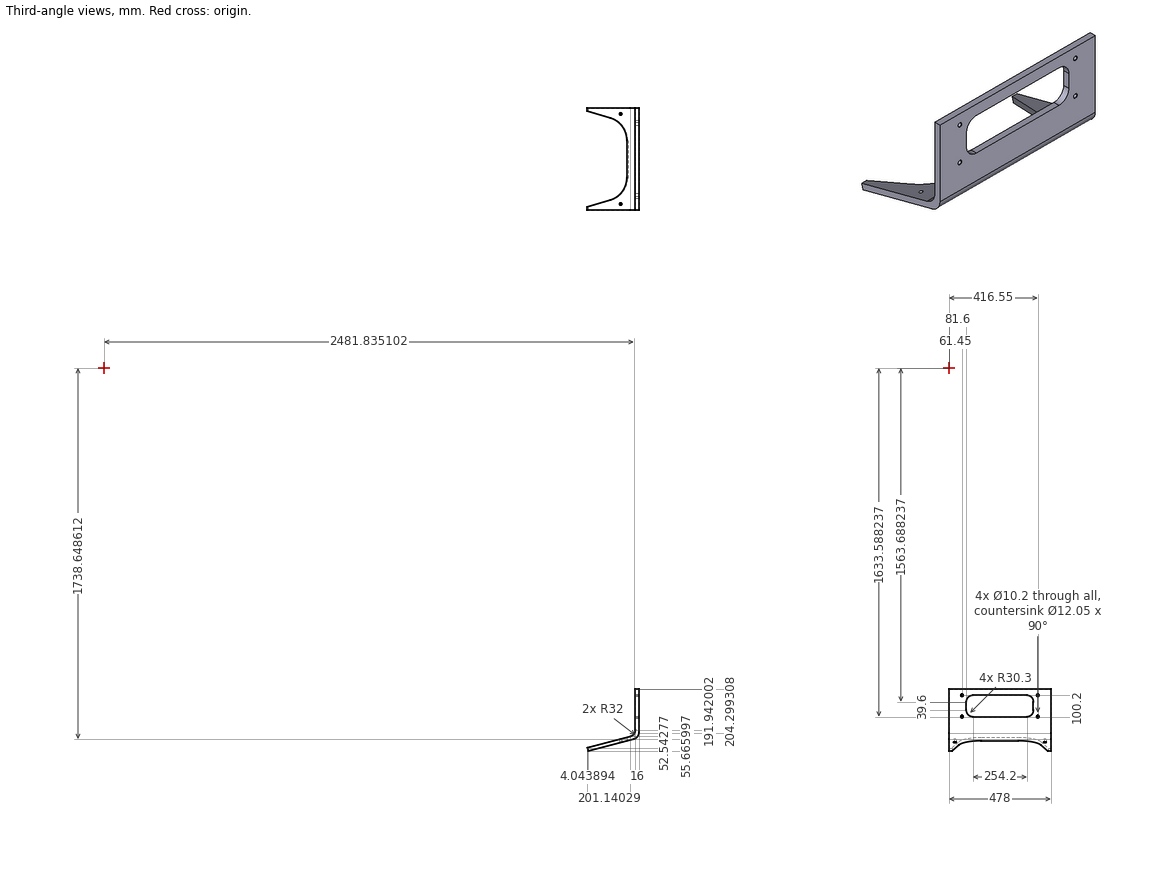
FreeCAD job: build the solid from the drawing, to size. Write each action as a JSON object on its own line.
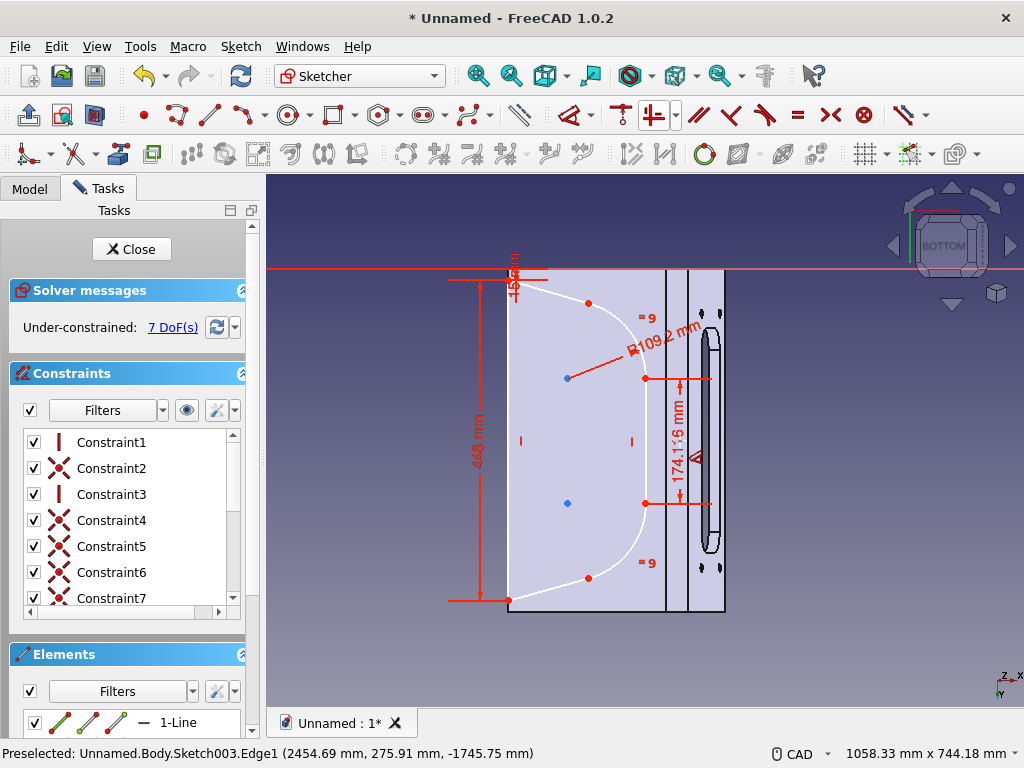
{"action": "left_click", "coordinate": [588, 303]}
{"action": "left_click", "coordinate": [622, 286]}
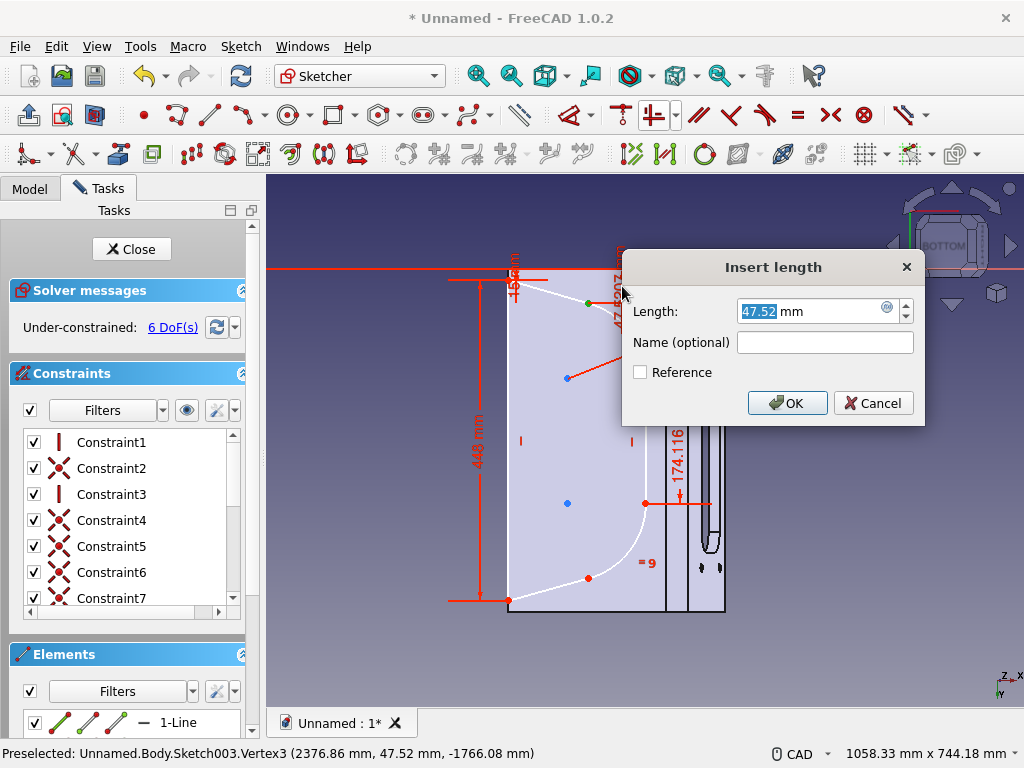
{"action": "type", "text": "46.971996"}
{"action": "key", "text": "Return"}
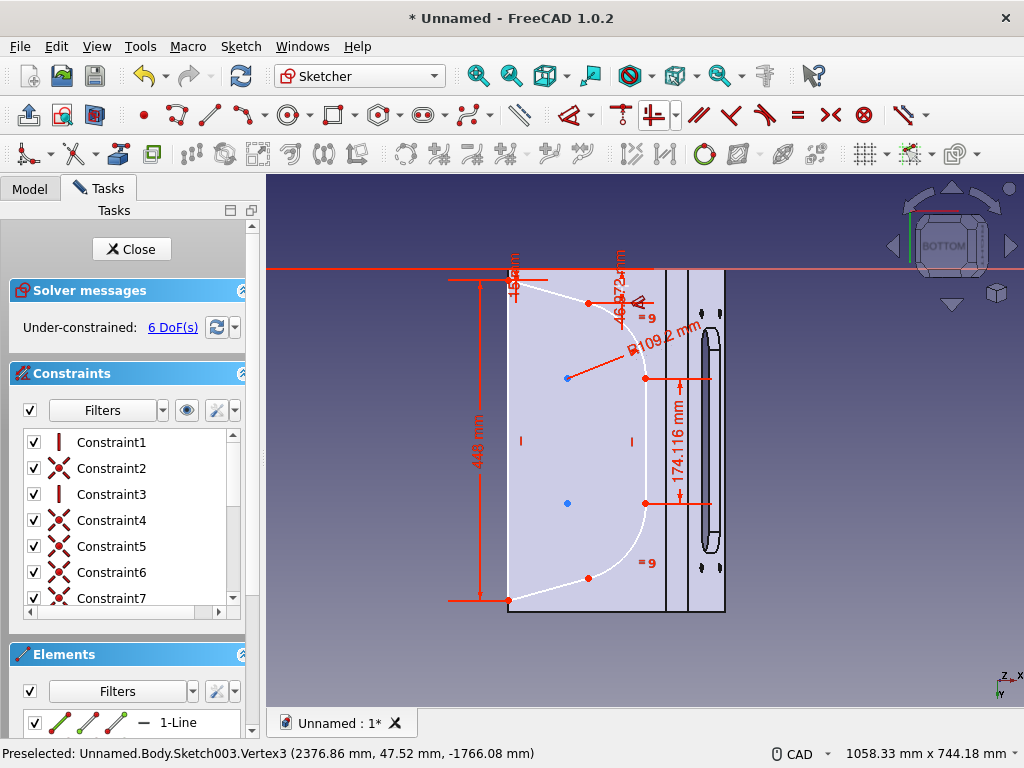
{"action": "scroll", "coordinate": [532, 594], "scroll_direction": "up", "scroll_amount": 3}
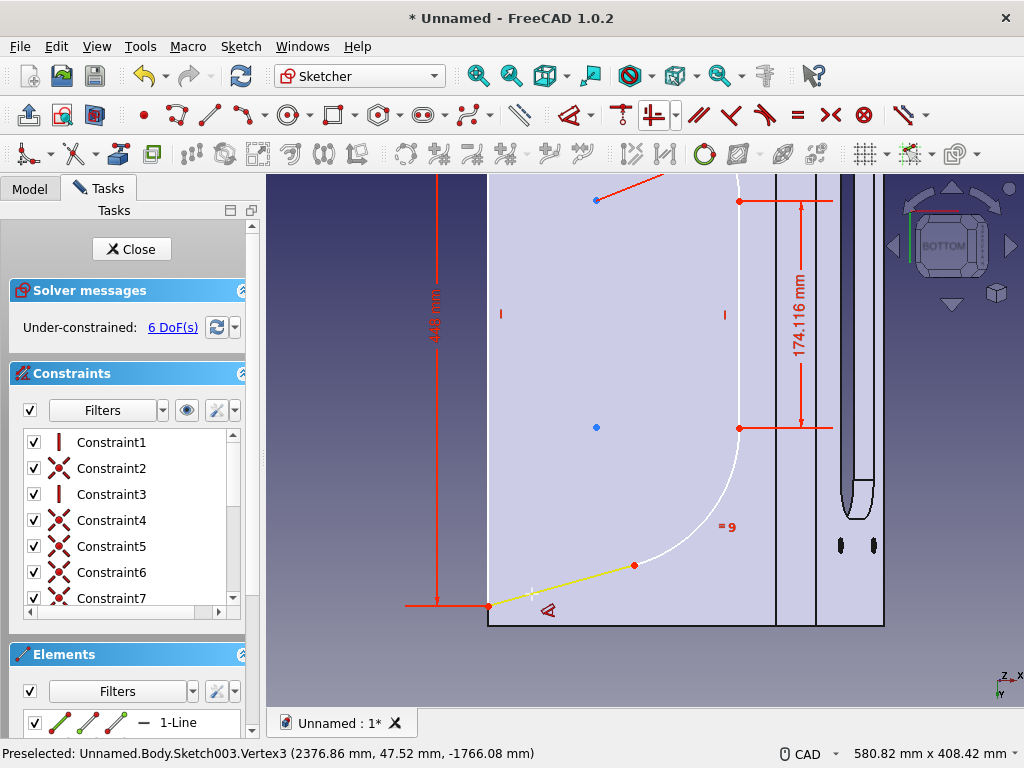
{"action": "left_click", "coordinate": [532, 594]}
{"action": "left_click", "coordinate": [454, 586]}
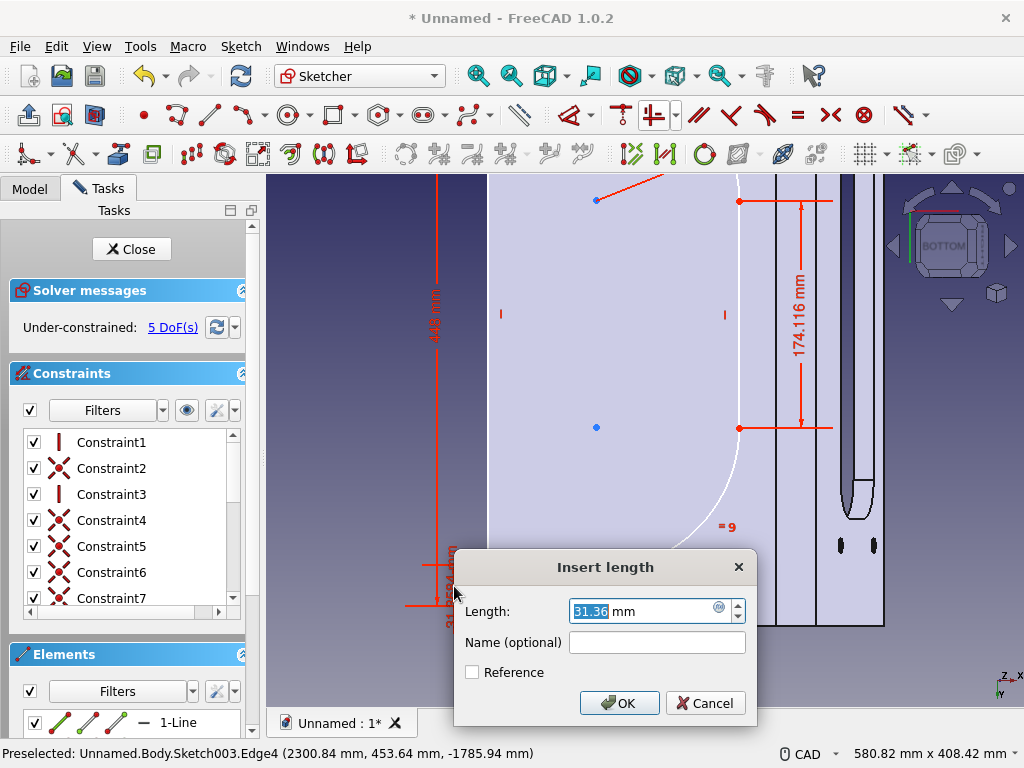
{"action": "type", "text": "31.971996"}
{"action": "key", "text": "Return"}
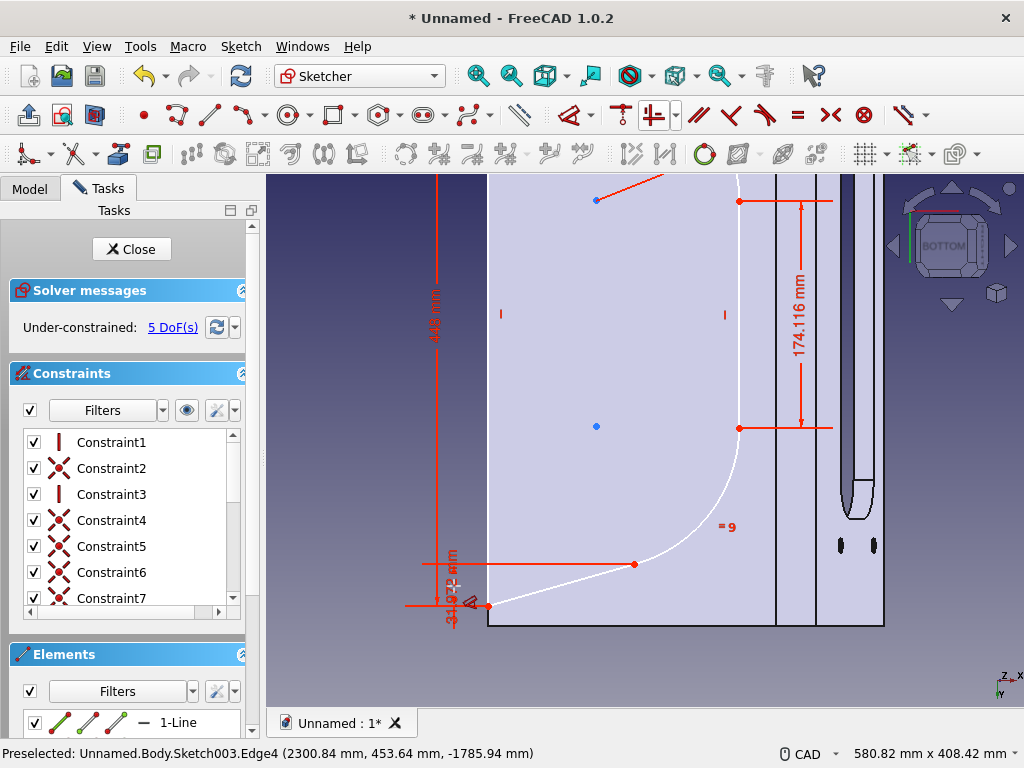
{"action": "left_click", "coordinate": [739, 428]}
{"action": "left_click", "coordinate": [773, 263]}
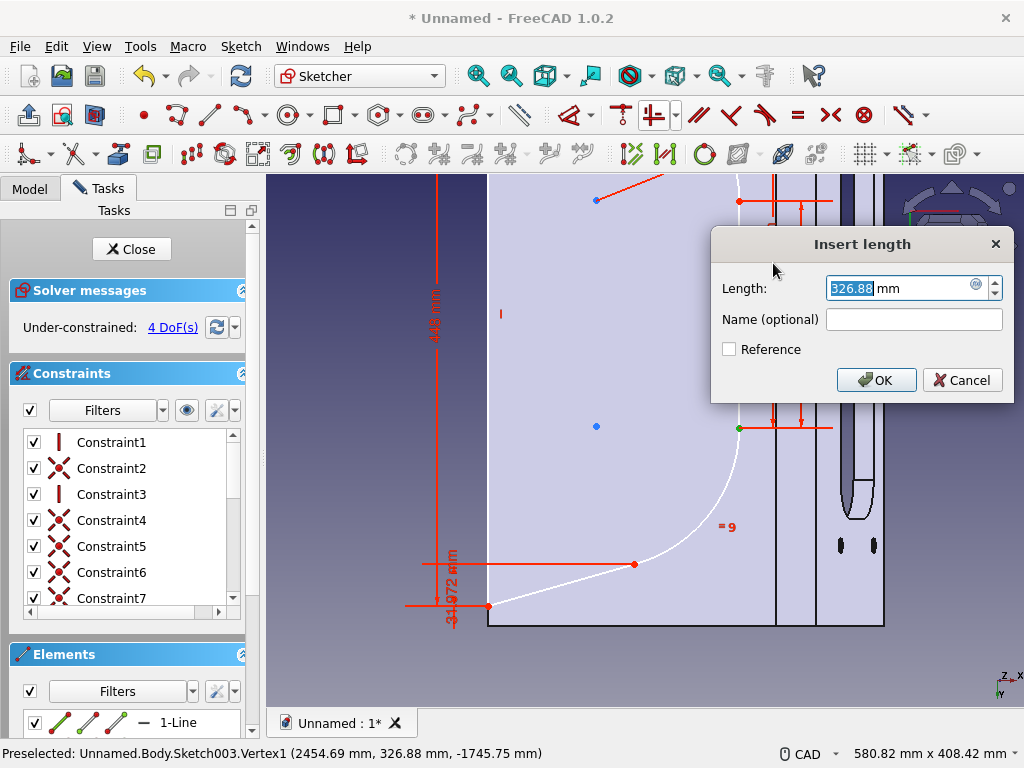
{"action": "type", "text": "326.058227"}
{"action": "key", "text": "Return"}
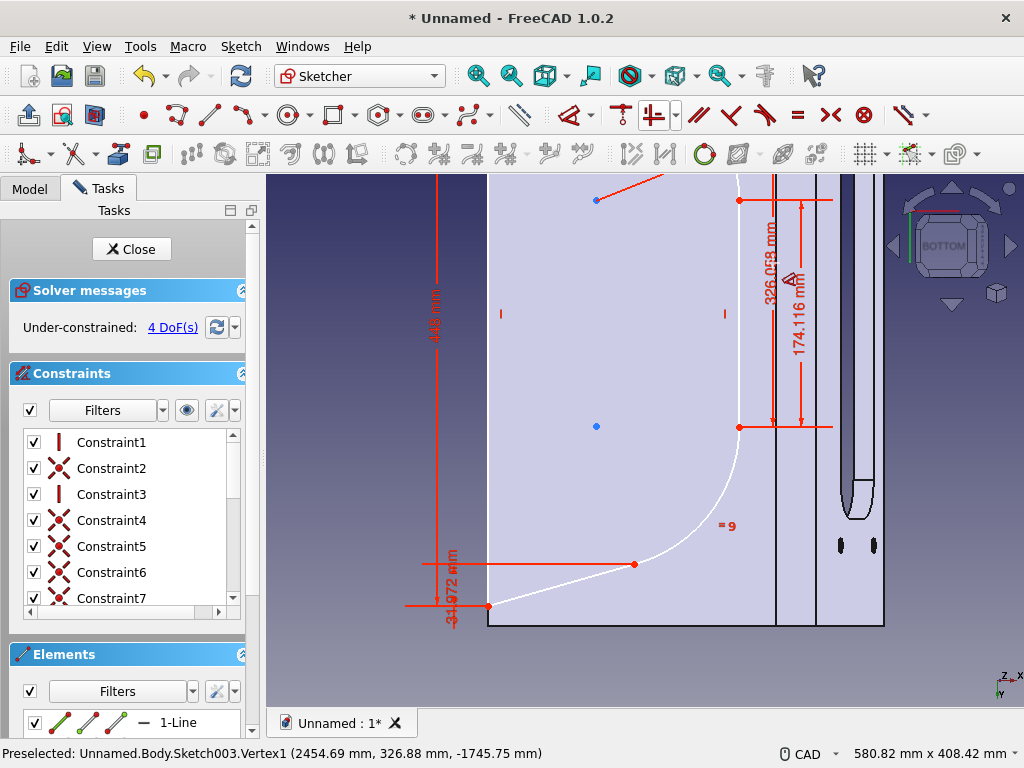
{"action": "scroll", "coordinate": [532, 595], "scroll_direction": "down", "scroll_amount": 3}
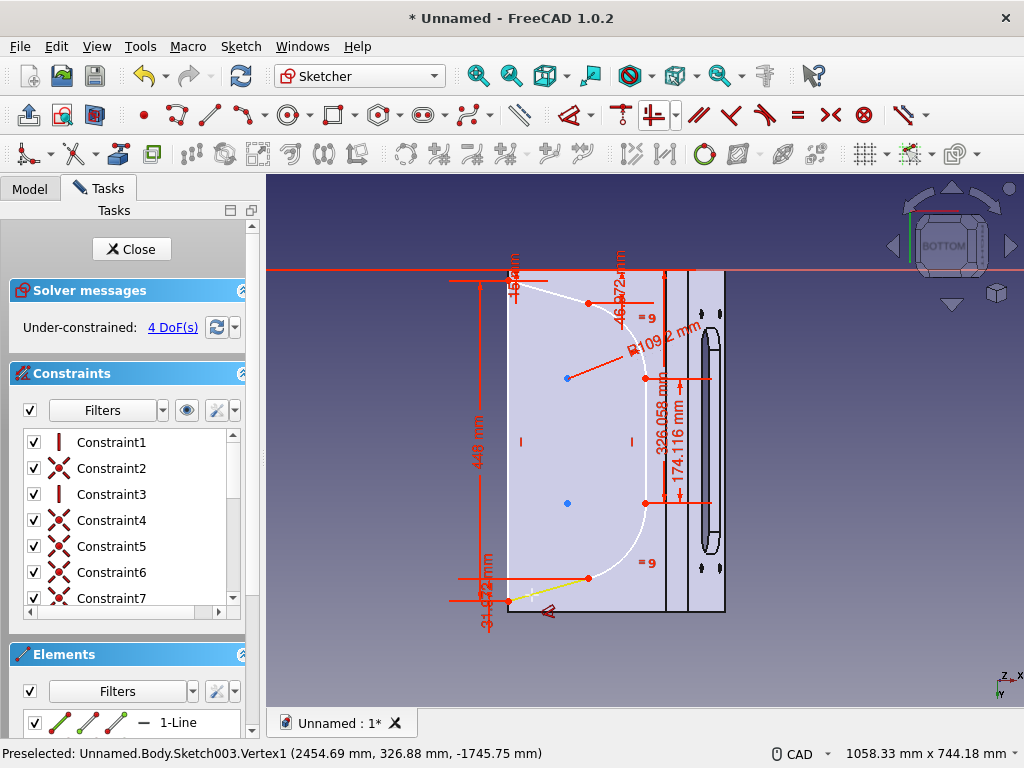
{"action": "left_click", "coordinate": [564, 297]}
{"action": "left_click", "coordinate": [548, 247]}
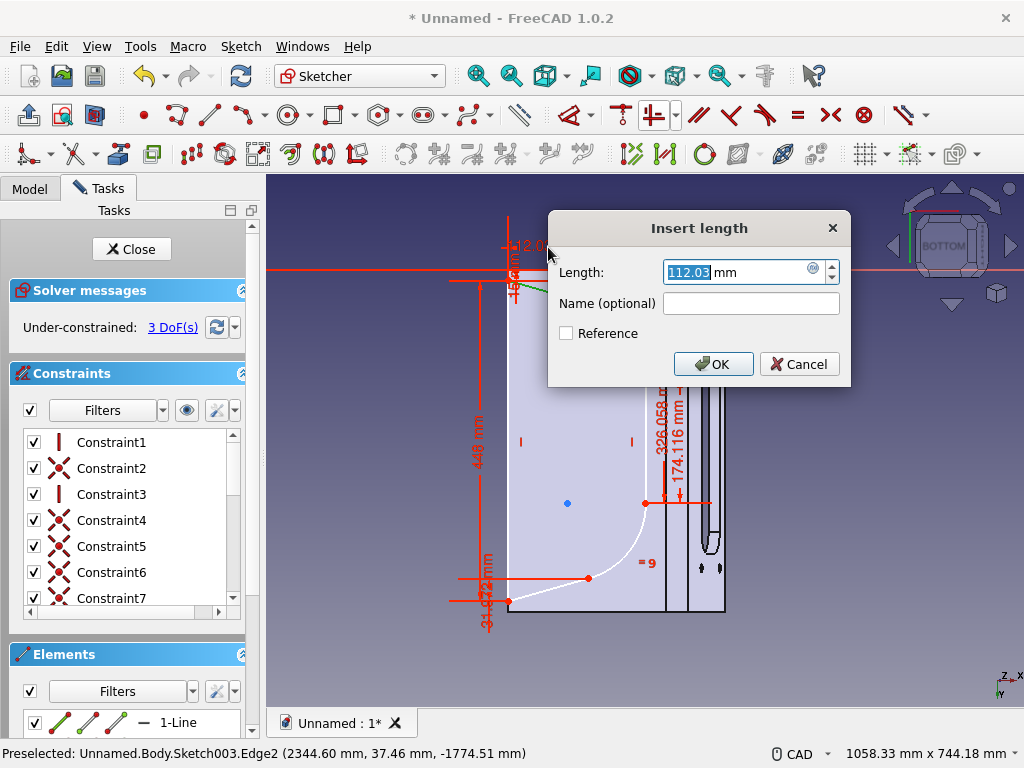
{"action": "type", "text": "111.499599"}
{"action": "key", "text": "Return"}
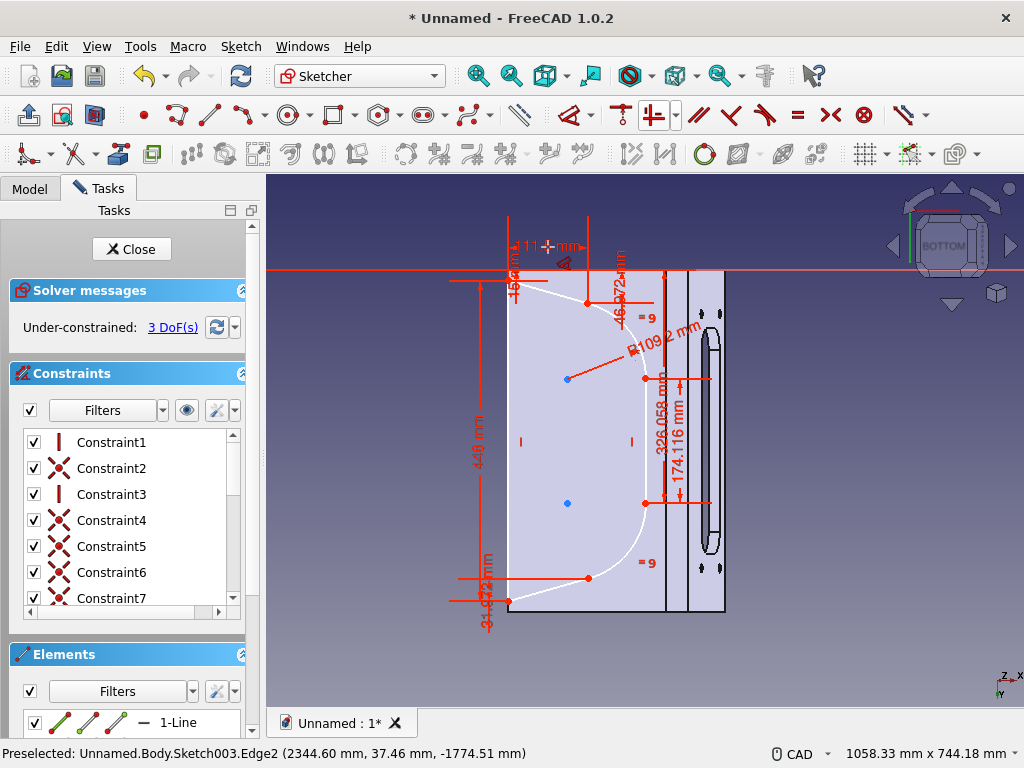
{"action": "left_click", "coordinate": [532, 595]}
{"action": "left_click", "coordinate": [548, 635]}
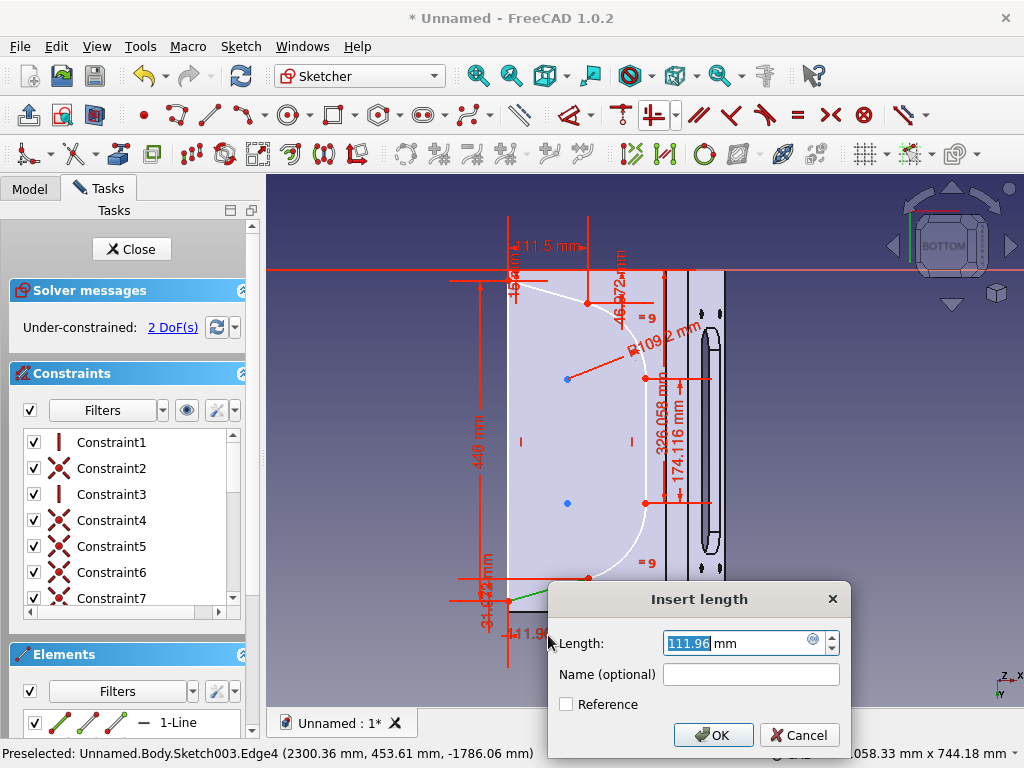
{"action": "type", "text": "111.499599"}
{"action": "key", "text": "Return"}